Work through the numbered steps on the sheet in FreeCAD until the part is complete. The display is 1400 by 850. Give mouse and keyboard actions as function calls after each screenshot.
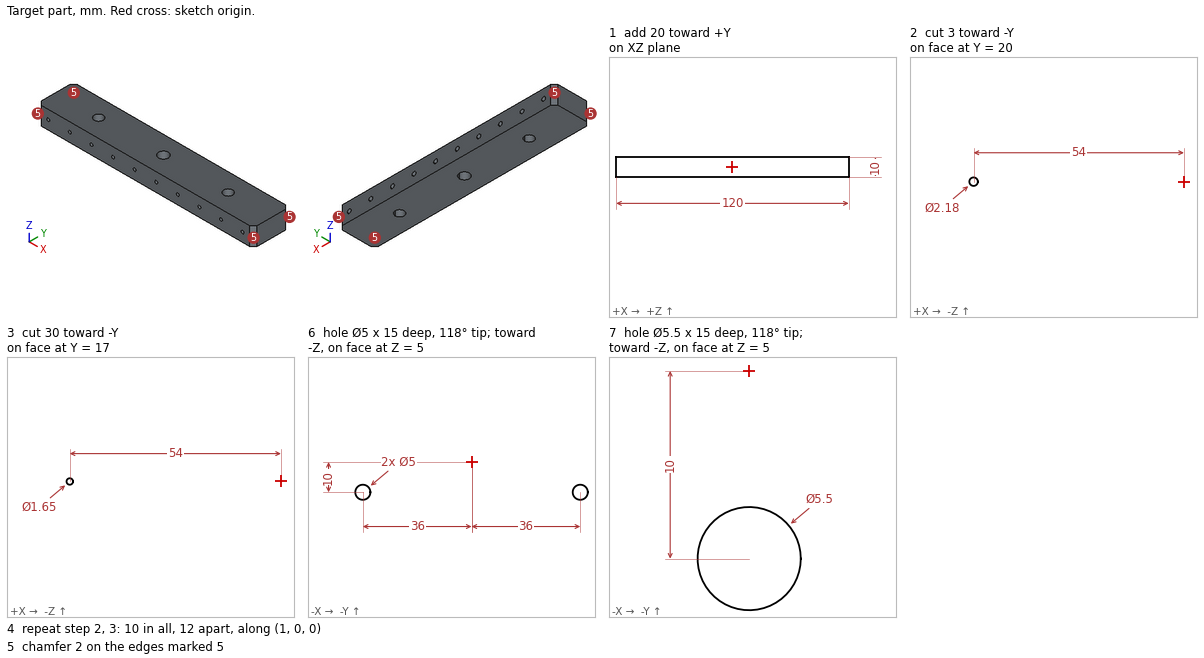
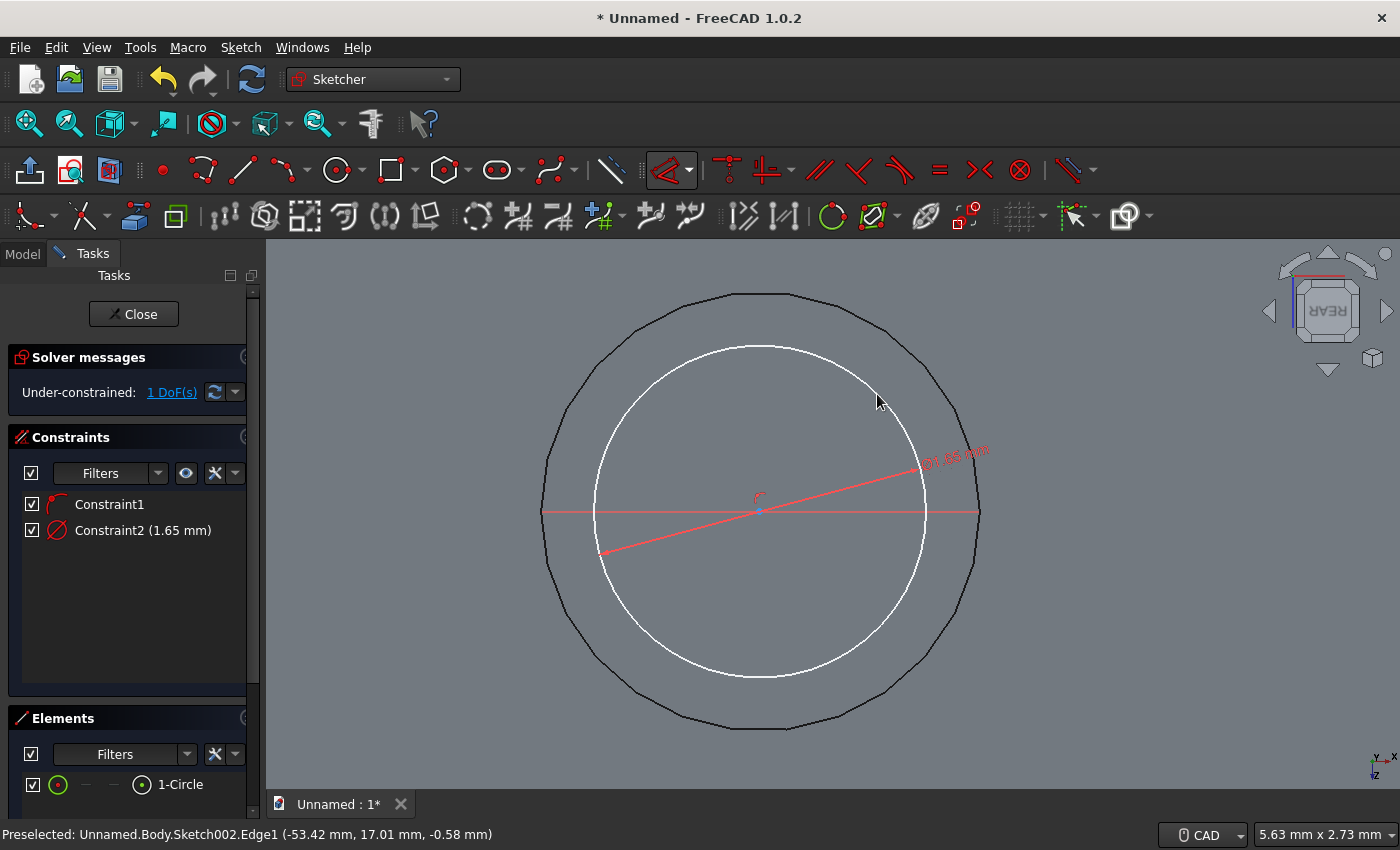
click(760, 512)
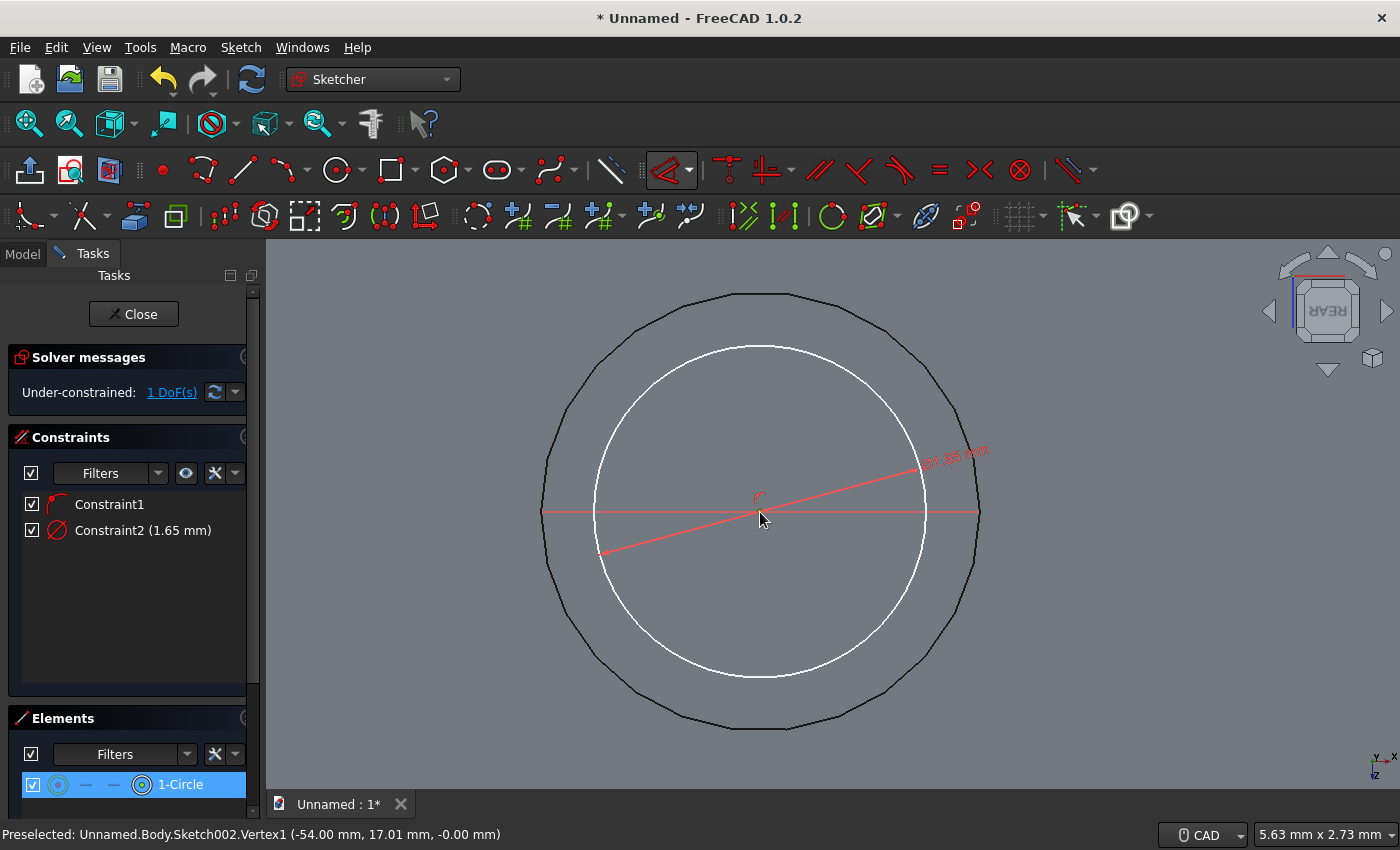
key(l)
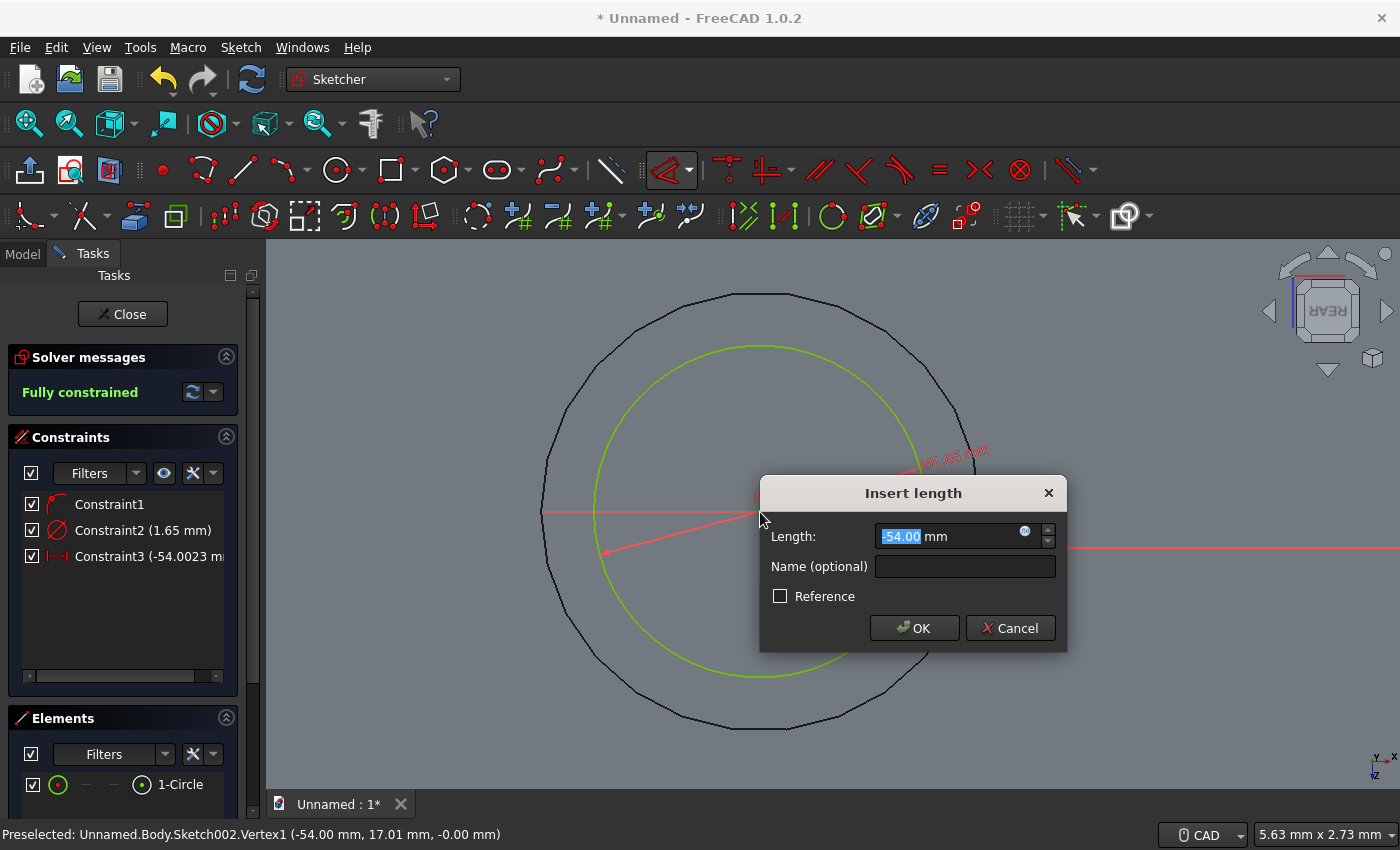
text(-54)
key(Return)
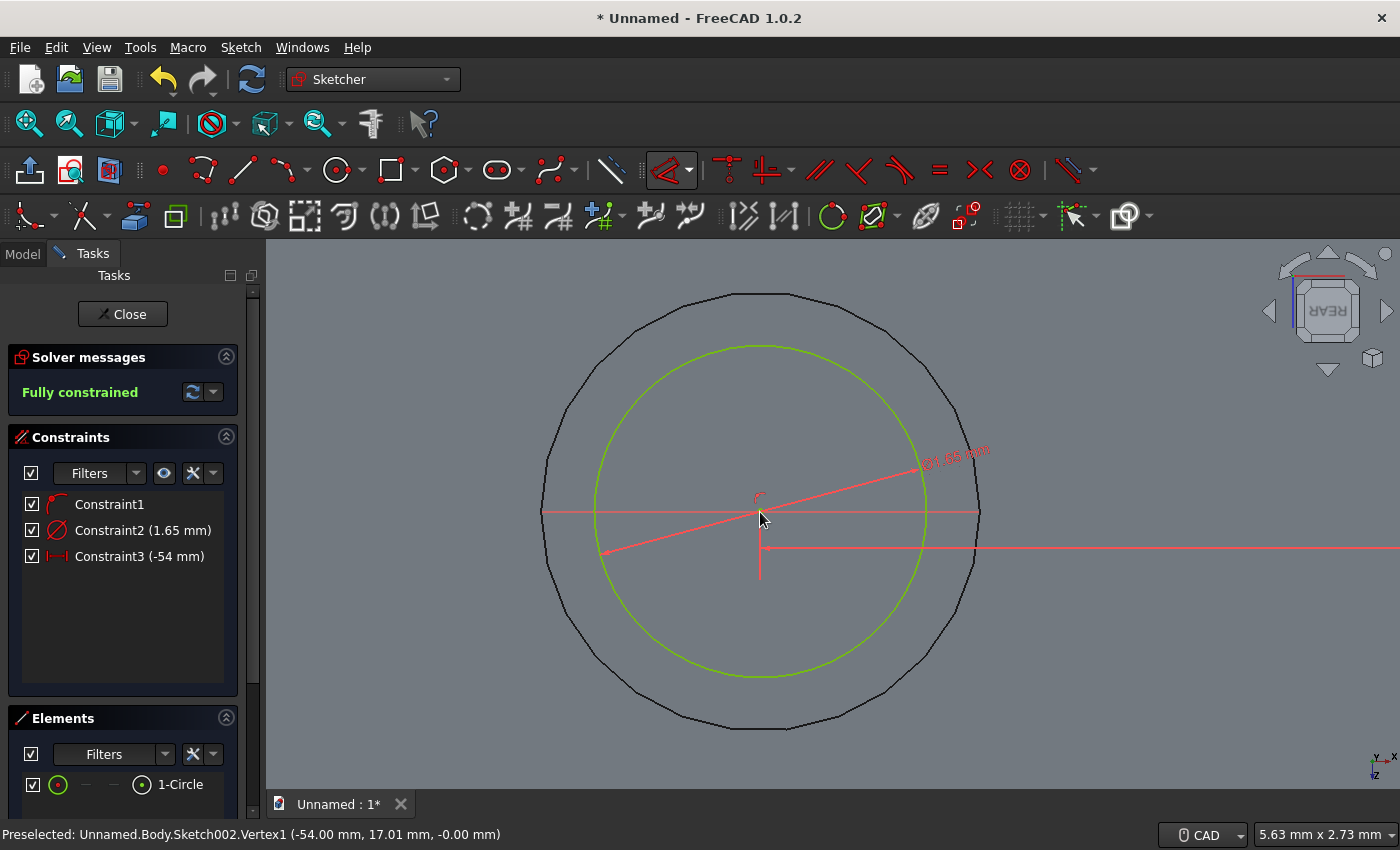
click(123, 314)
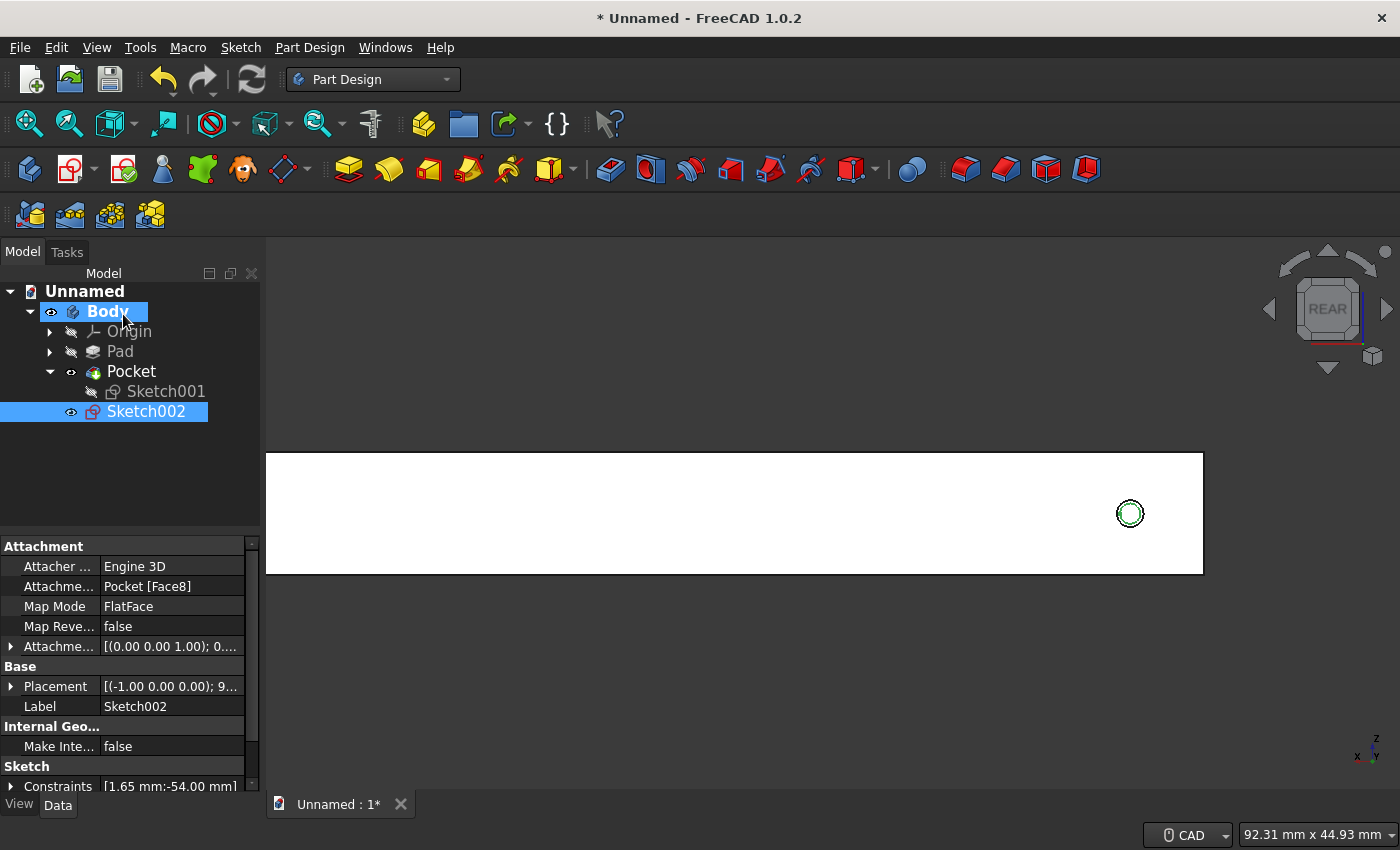
click(612, 170)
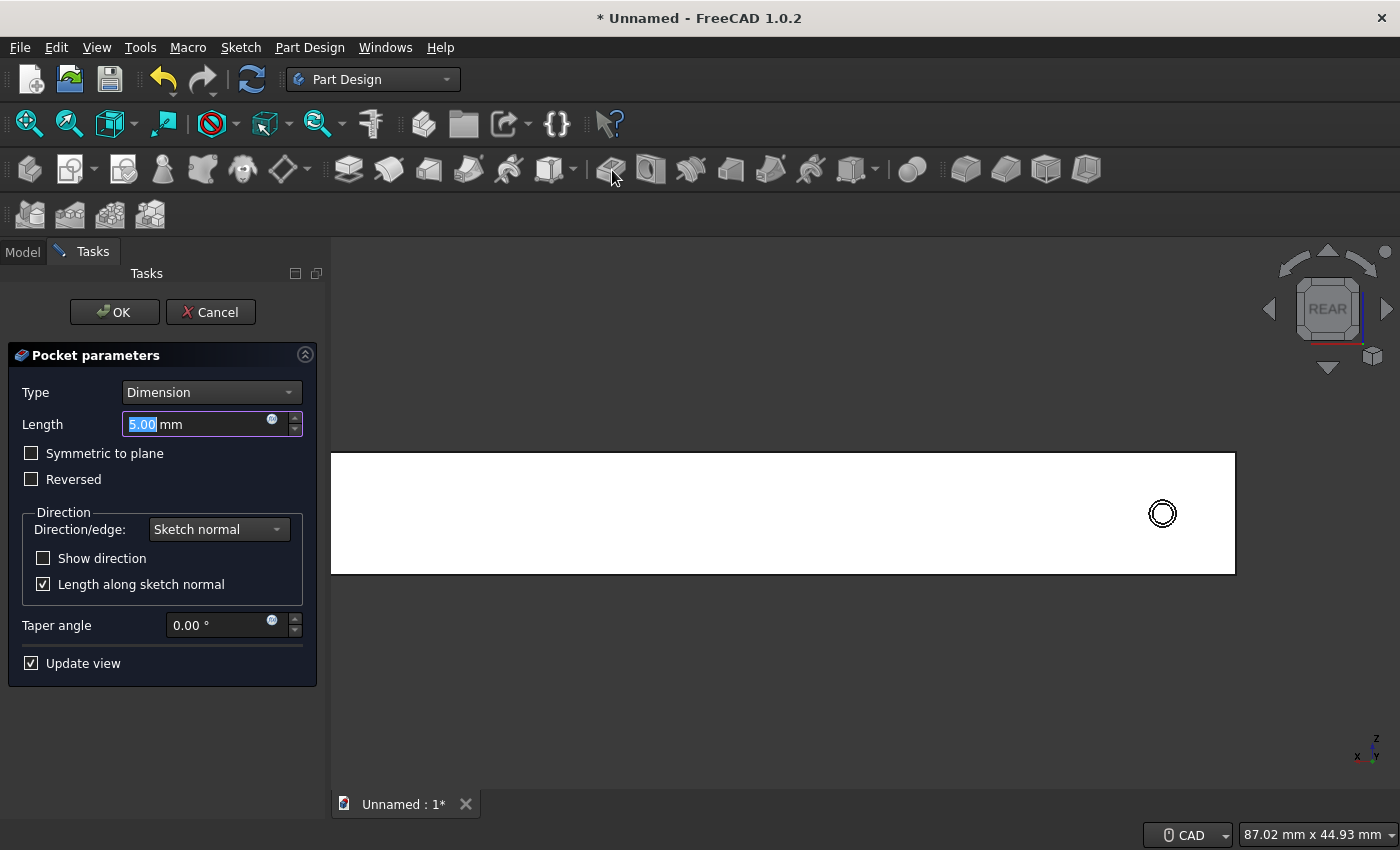
text(30)
key(Tab)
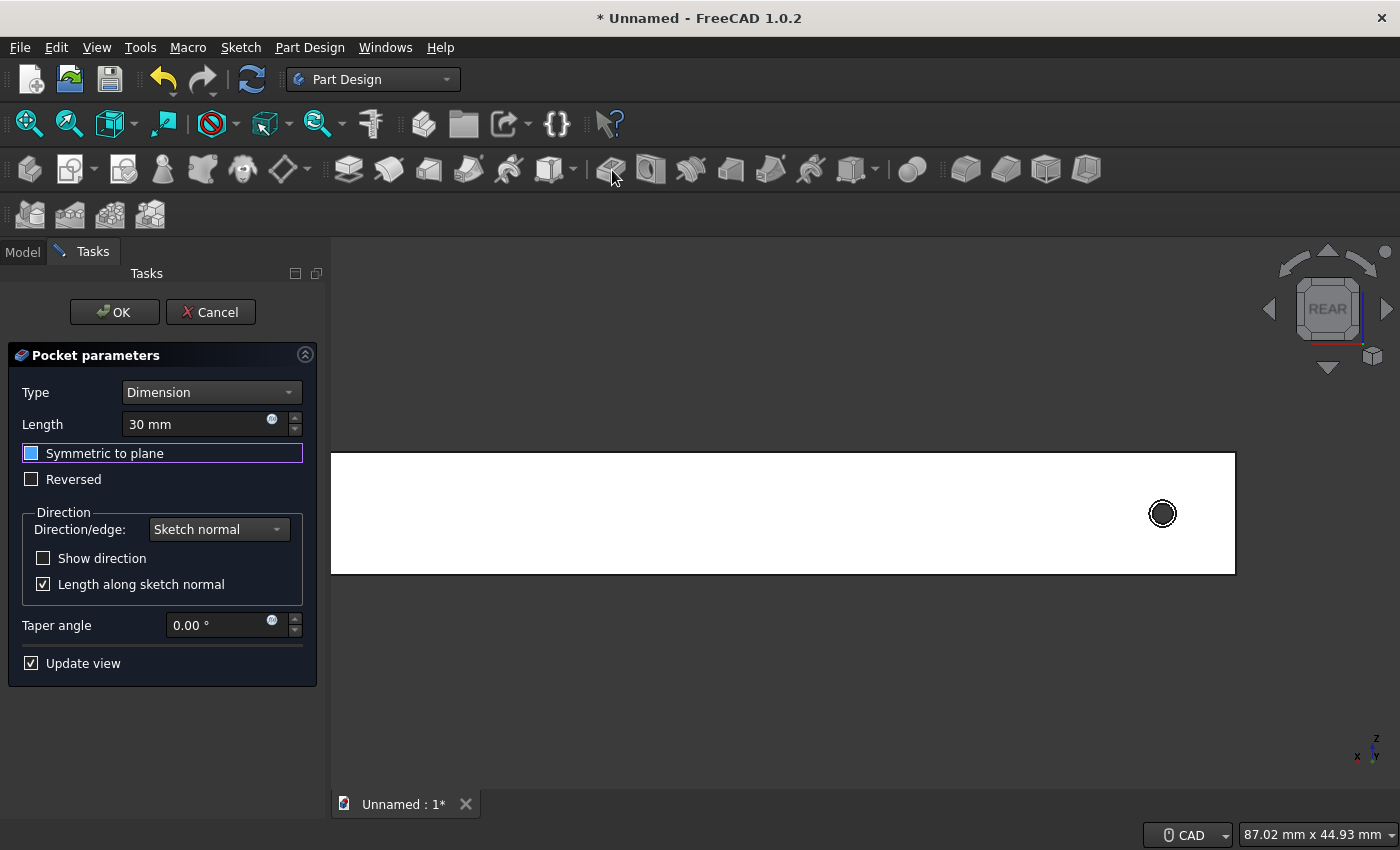
click(115, 312)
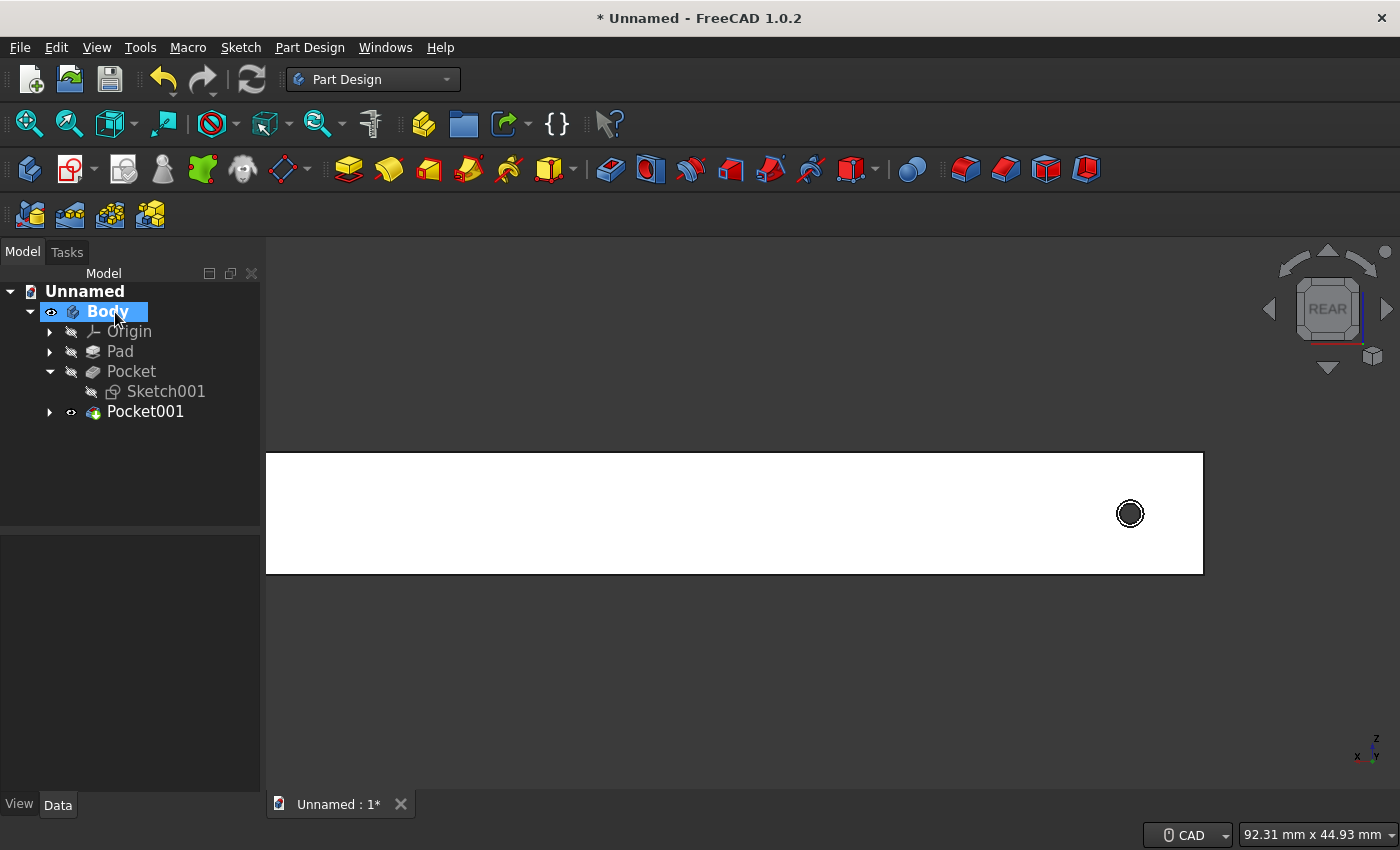
click(30, 124)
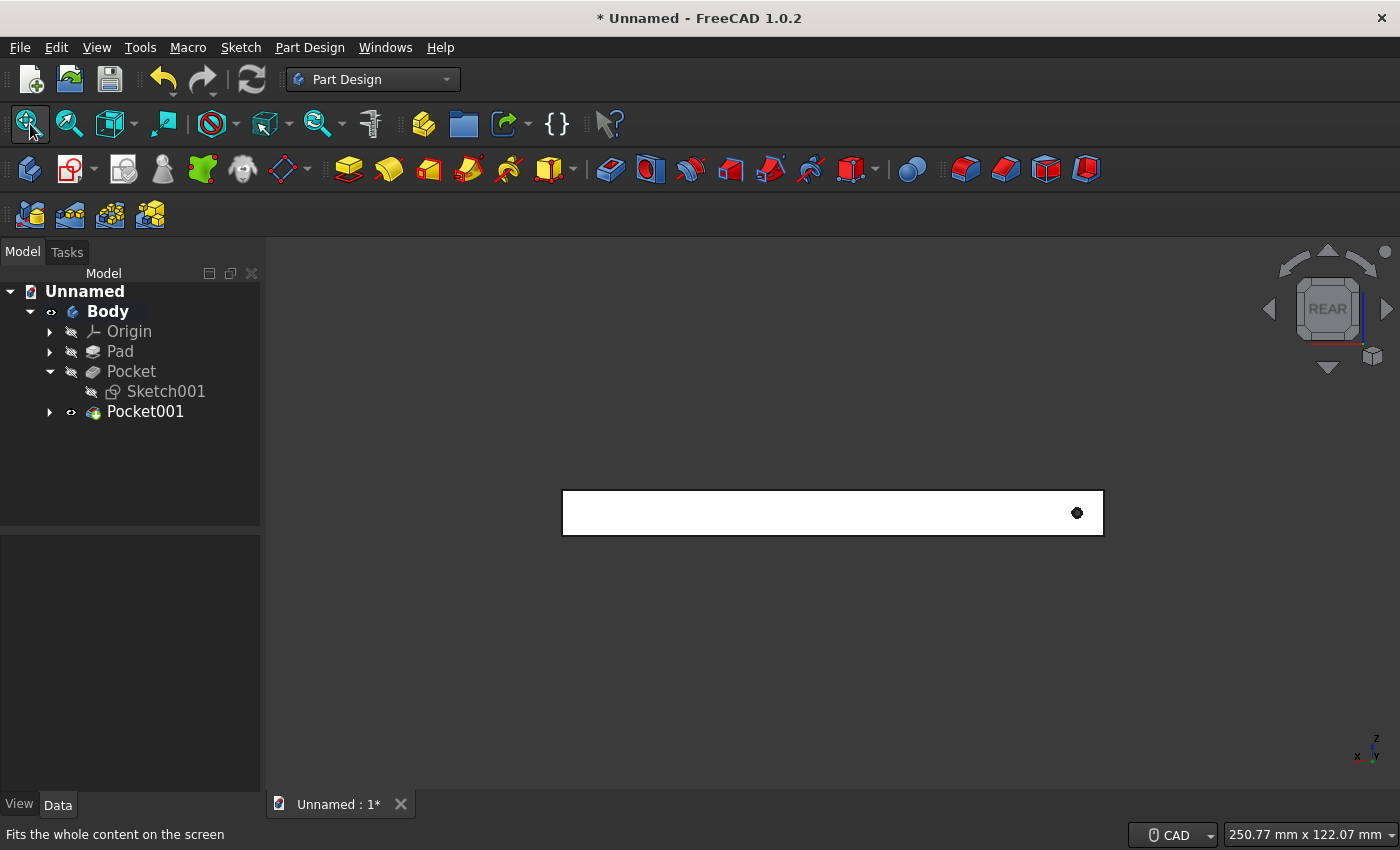
click(116, 372)